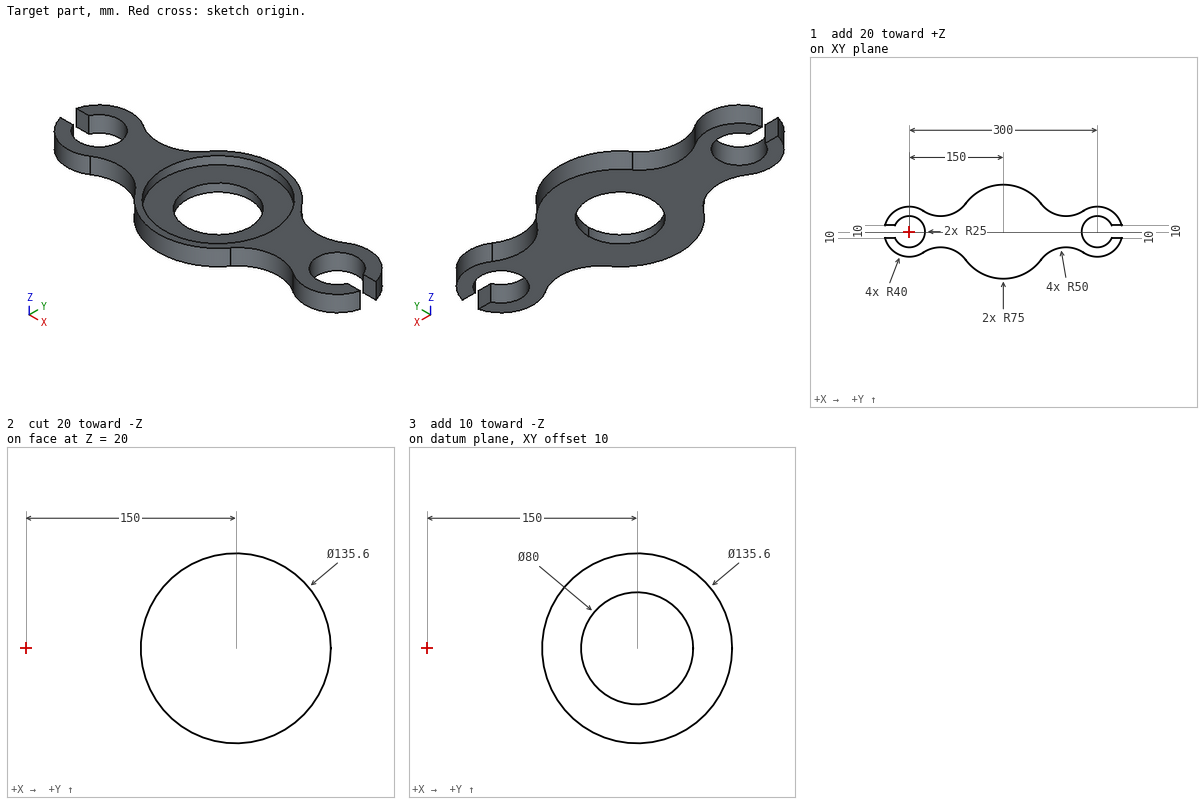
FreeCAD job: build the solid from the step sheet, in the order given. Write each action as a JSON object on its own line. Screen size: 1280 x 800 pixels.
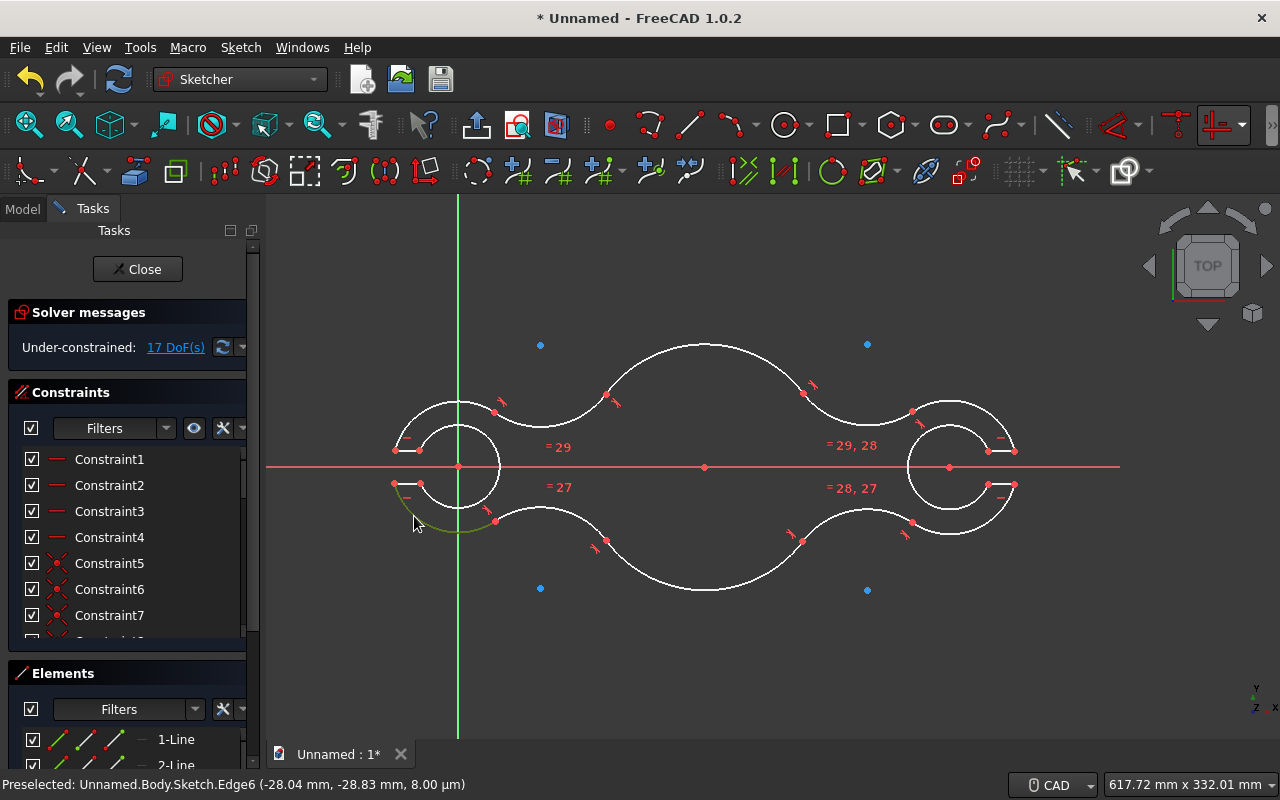
{"action": "left_click", "coordinate": [949, 534]}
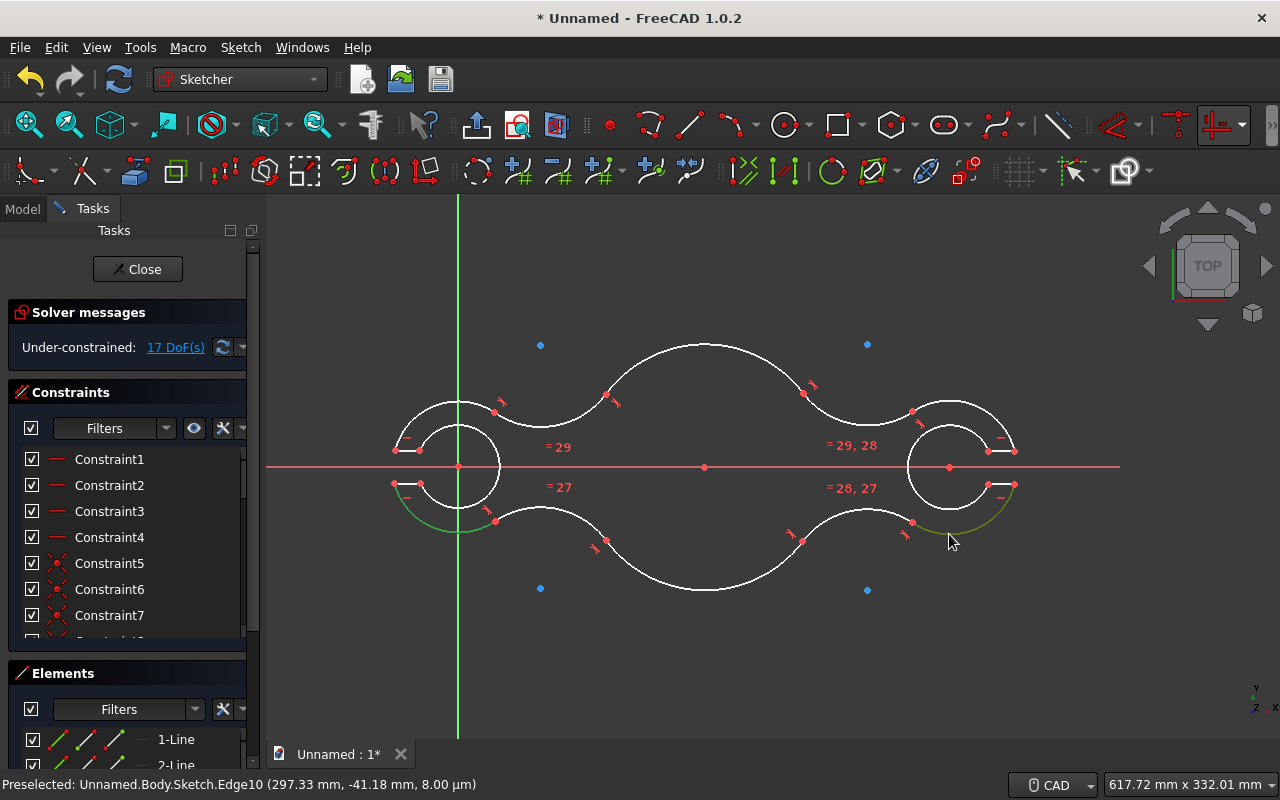
{"action": "left_click", "coordinate": [995, 419]}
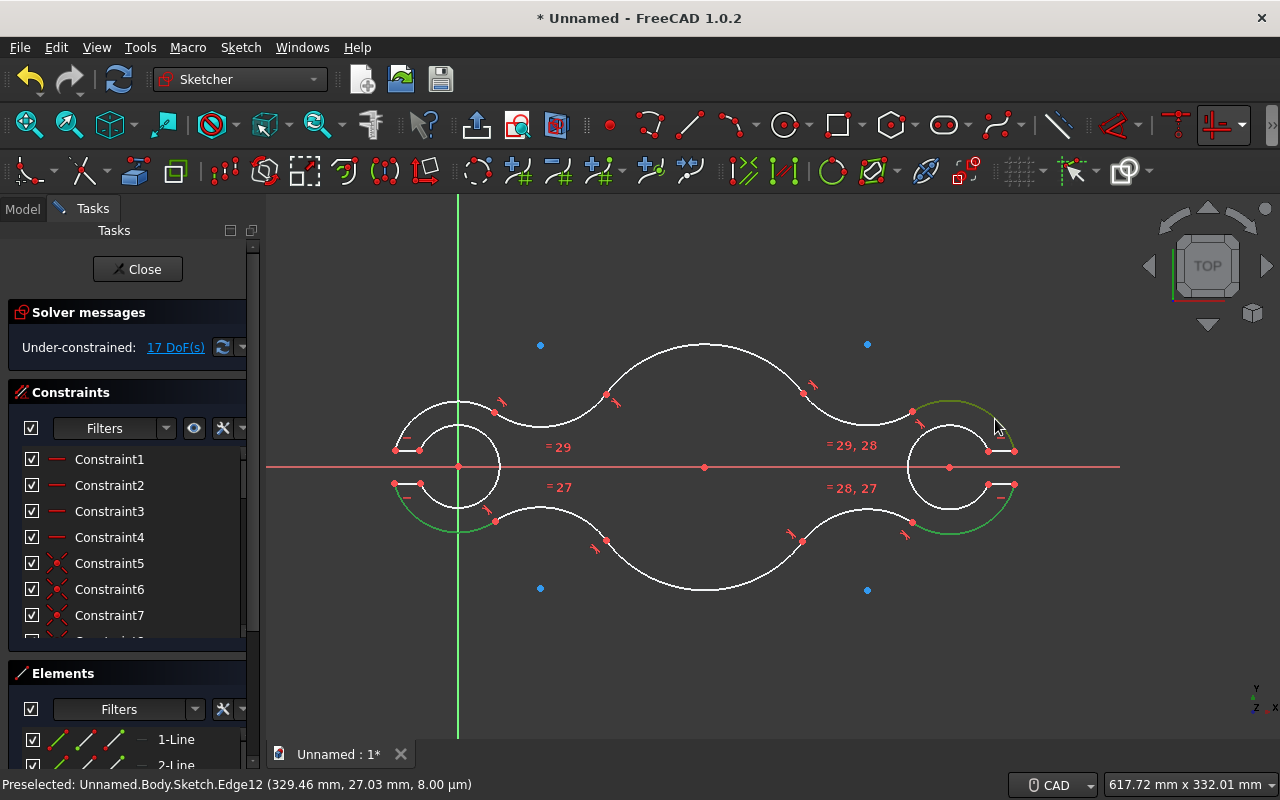
{"action": "left_click", "coordinate": [460, 401]}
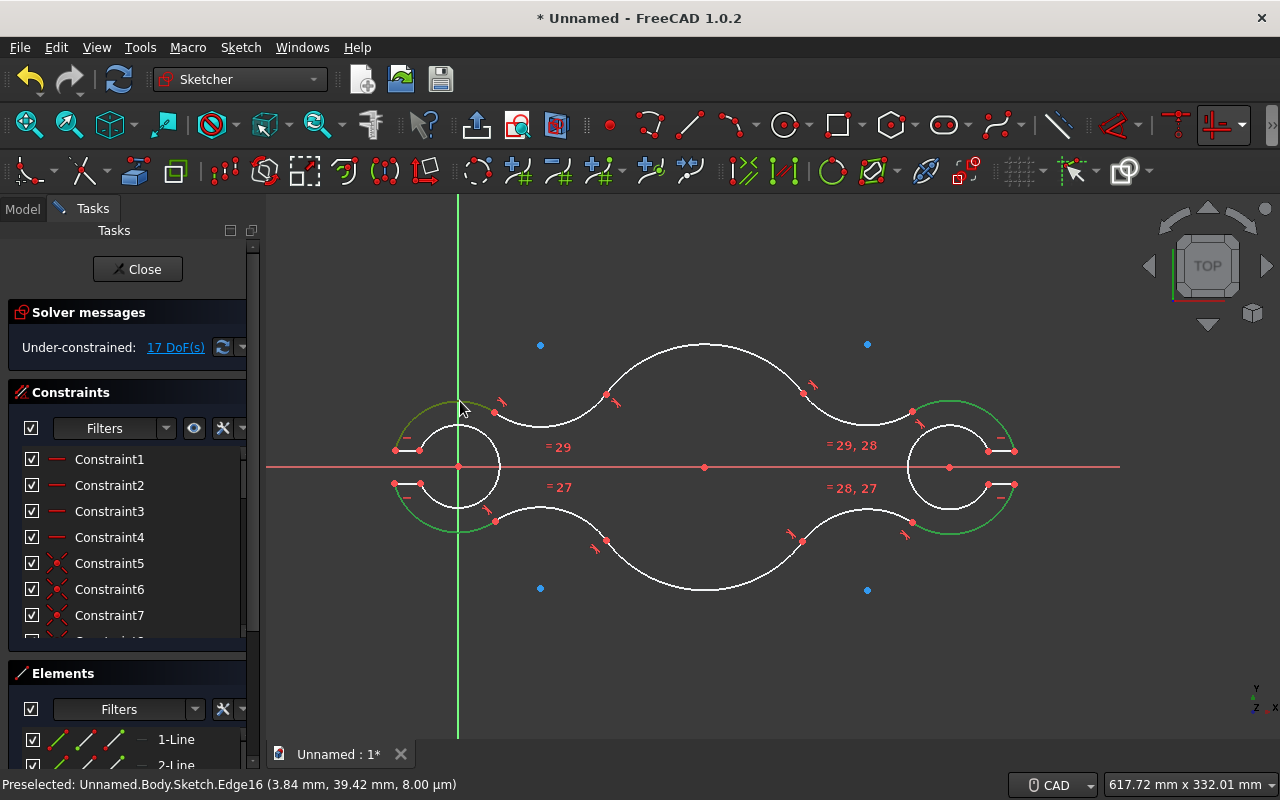
{"action": "key", "text": "e"}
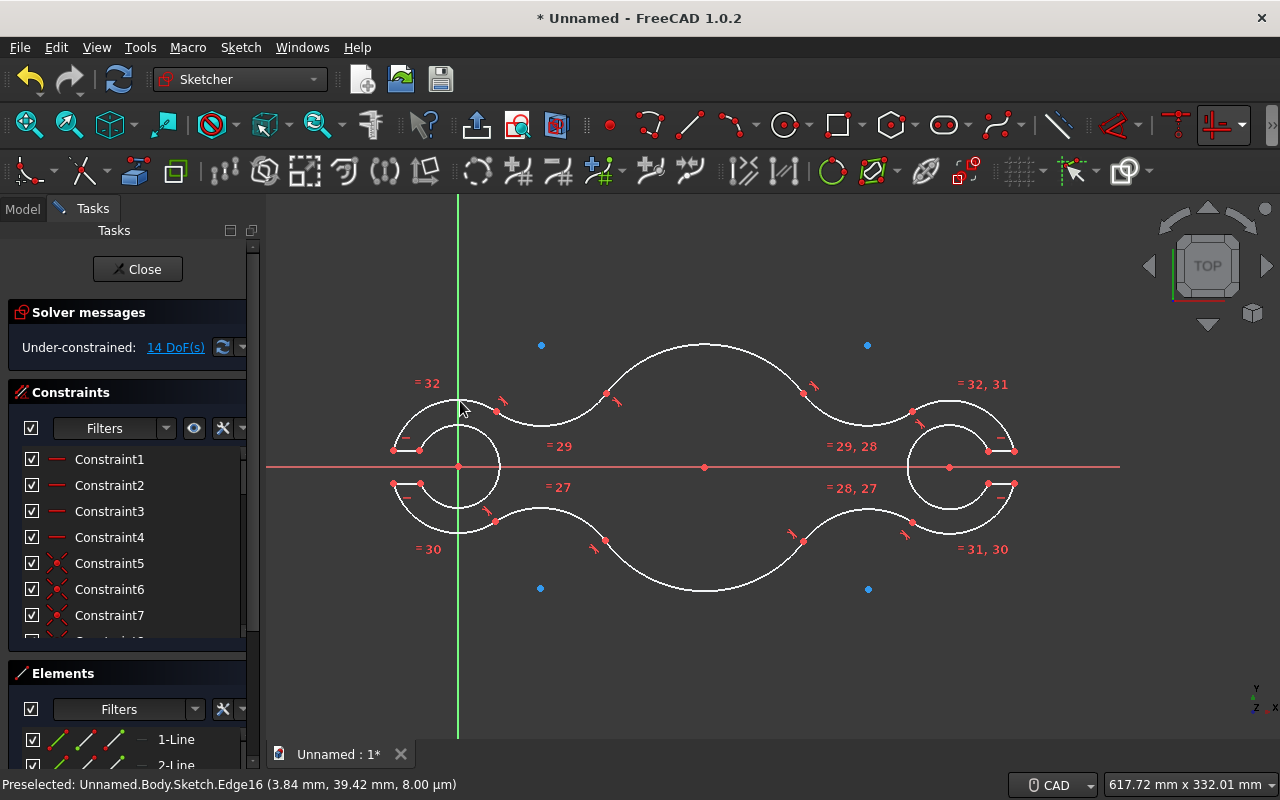
{"action": "left_click", "coordinate": [478, 503]}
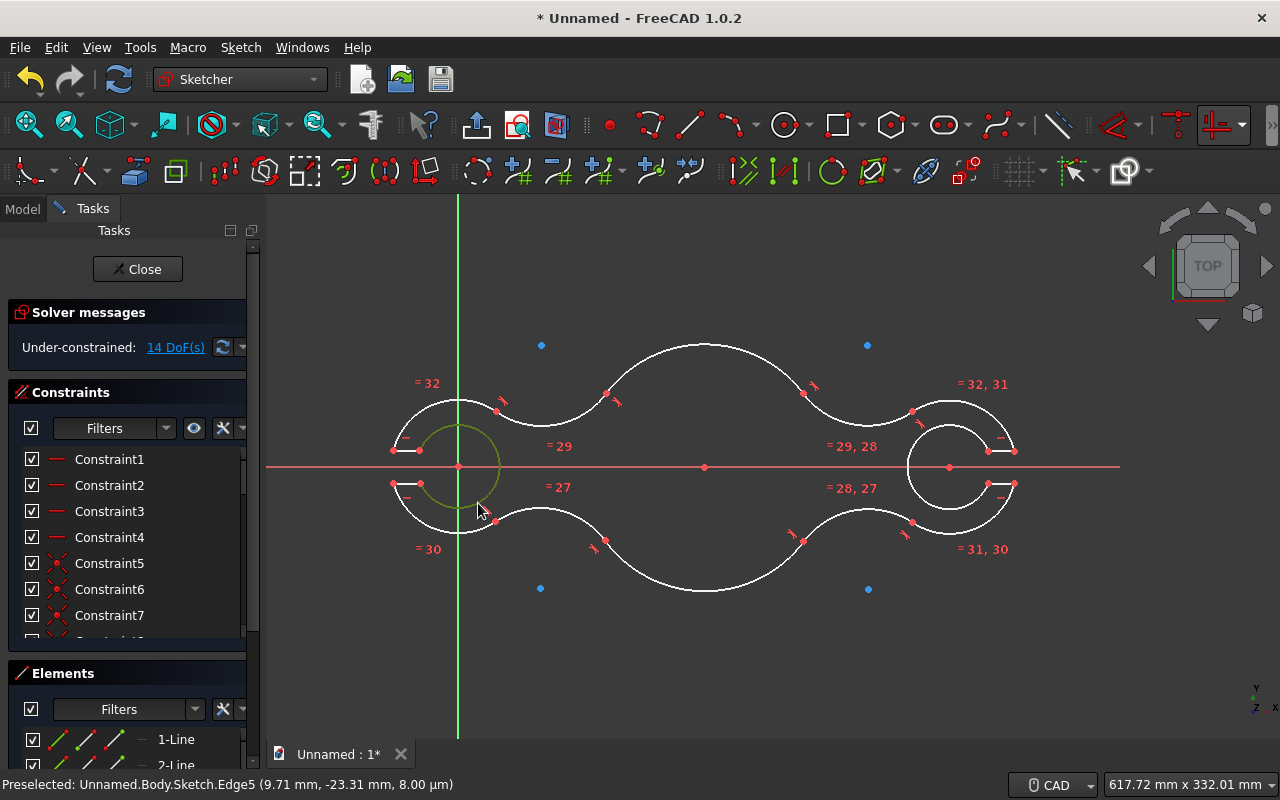
{"action": "left_click", "coordinate": [931, 430]}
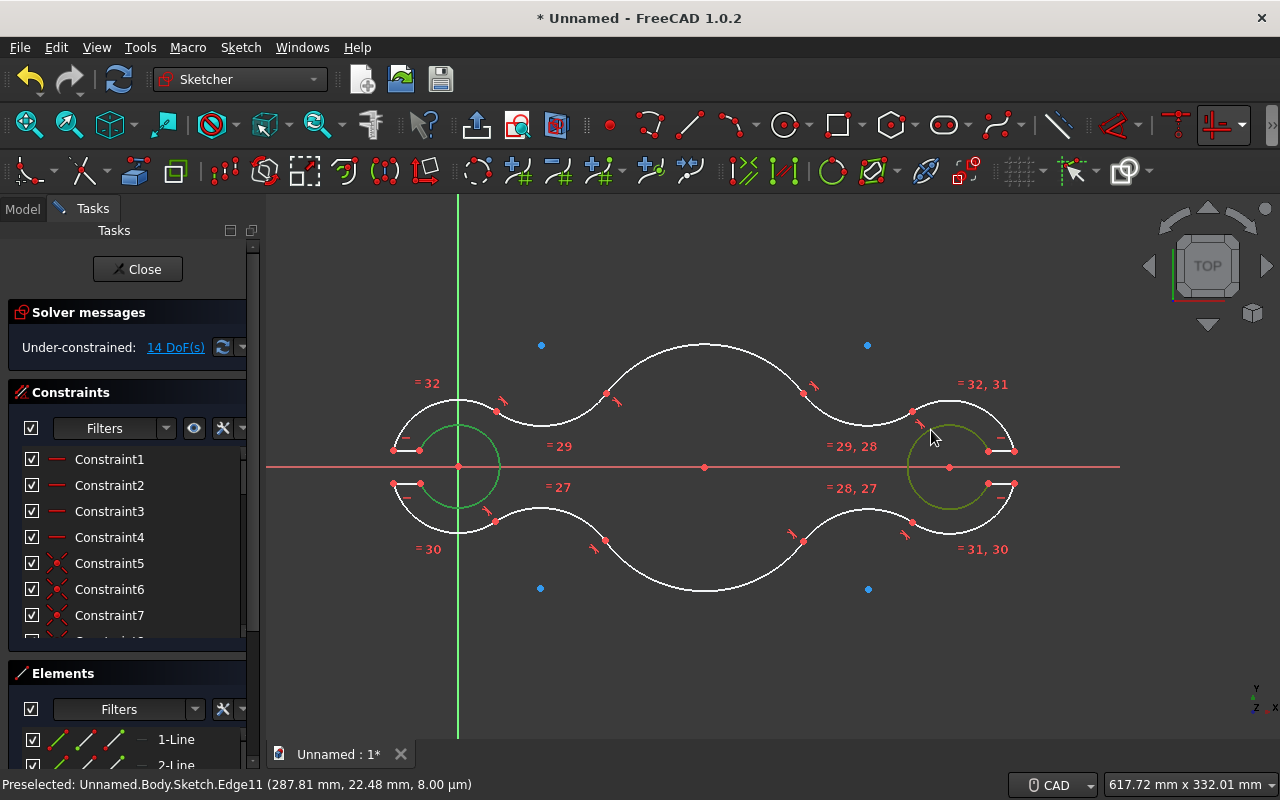
{"action": "key", "text": "e"}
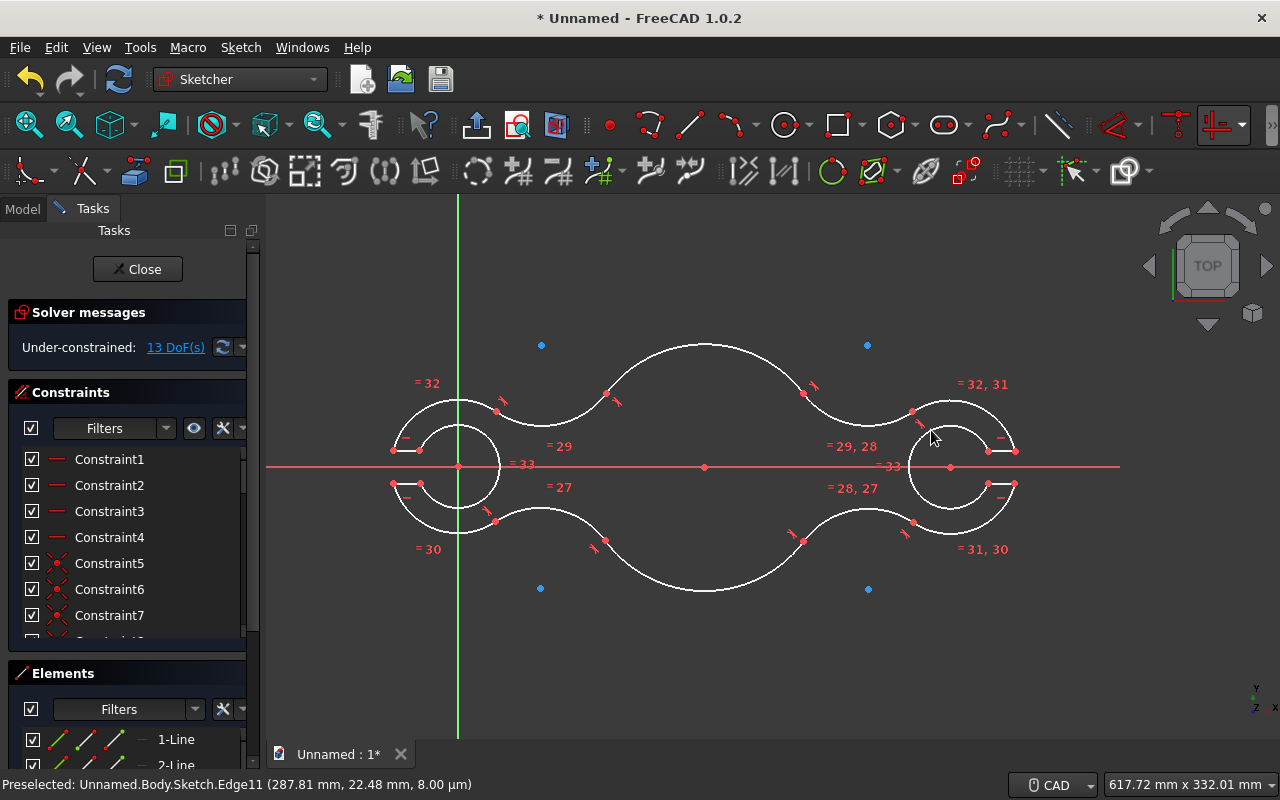
{"action": "left_click", "coordinate": [659, 582]}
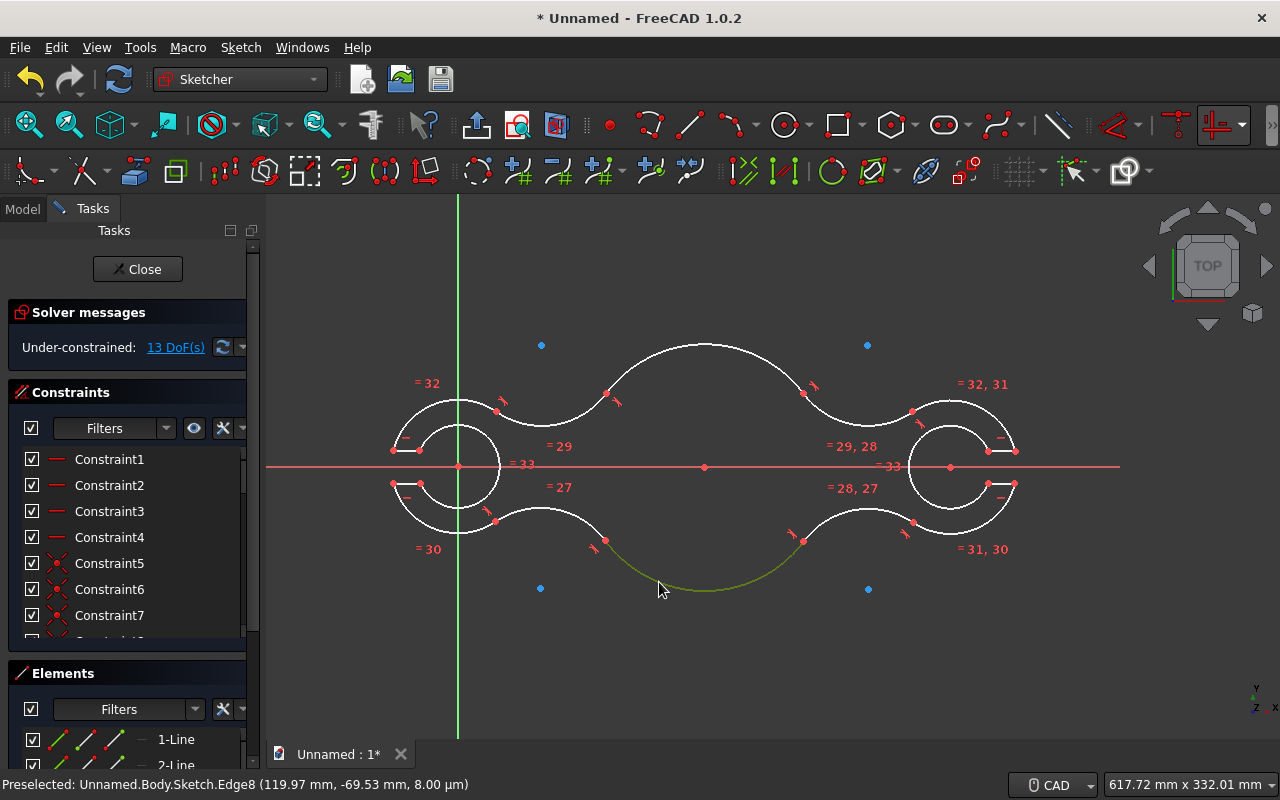
{"action": "left_click", "coordinate": [750, 353]}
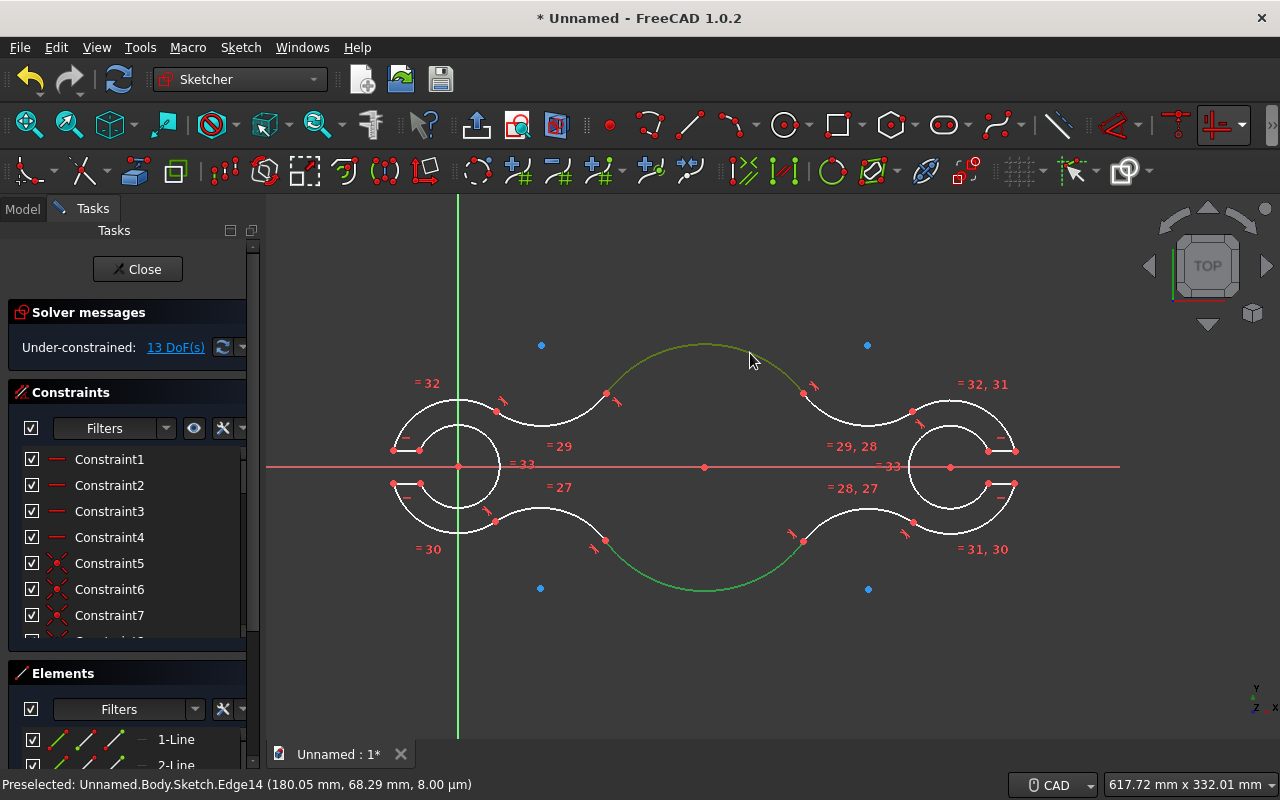
{"action": "key", "text": "e"}